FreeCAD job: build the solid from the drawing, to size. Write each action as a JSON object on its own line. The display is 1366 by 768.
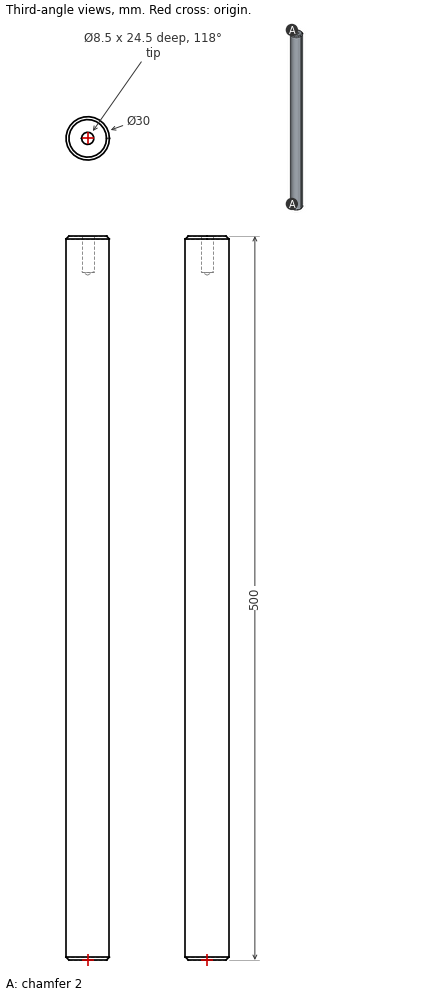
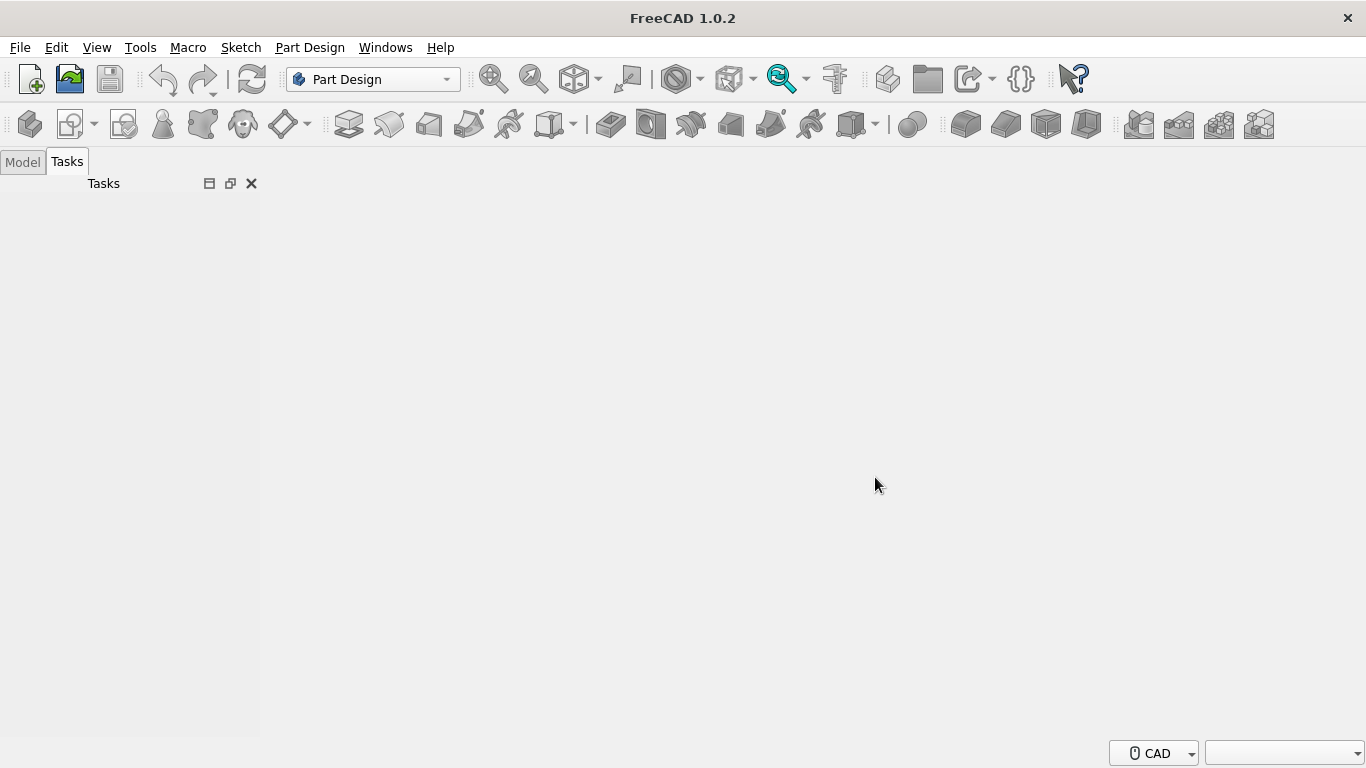
{"action": "left_click", "coordinate": [30, 80]}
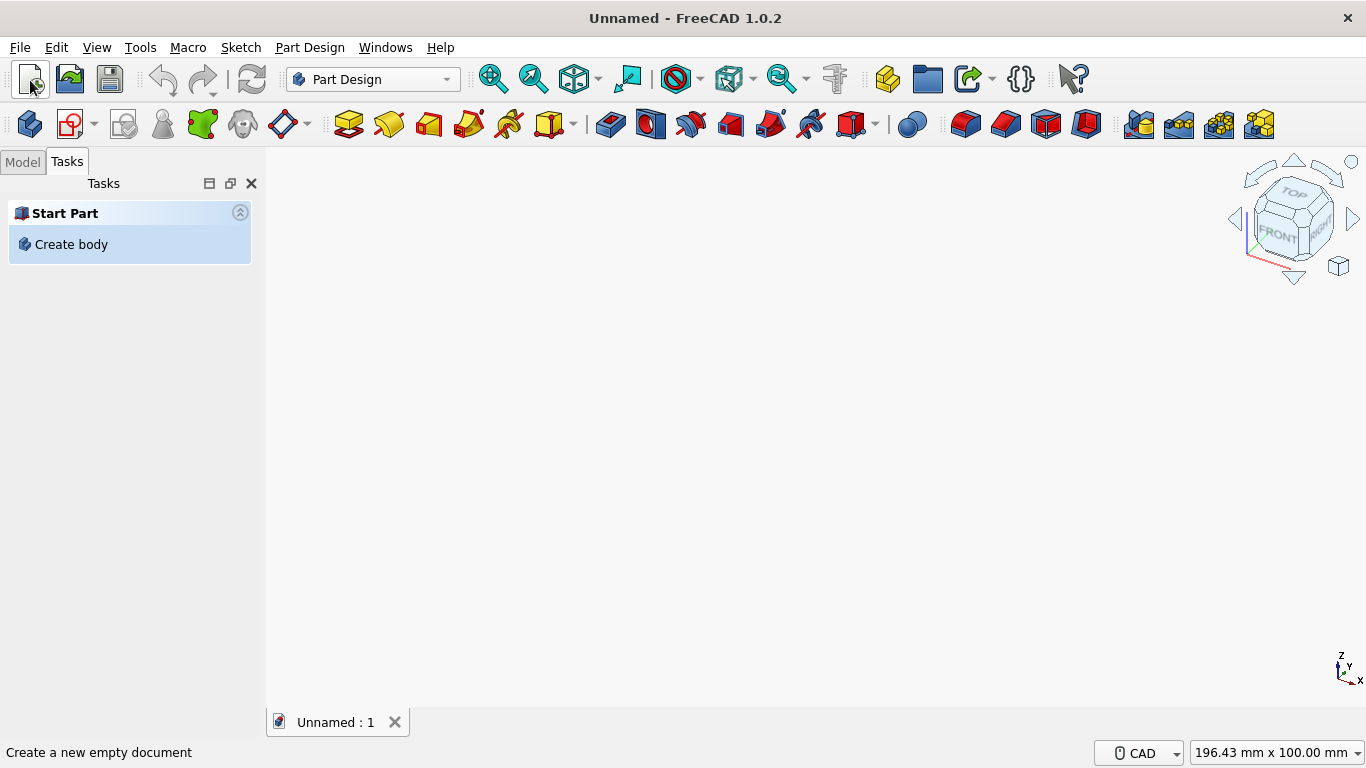
{"action": "left_click", "coordinate": [70, 124]}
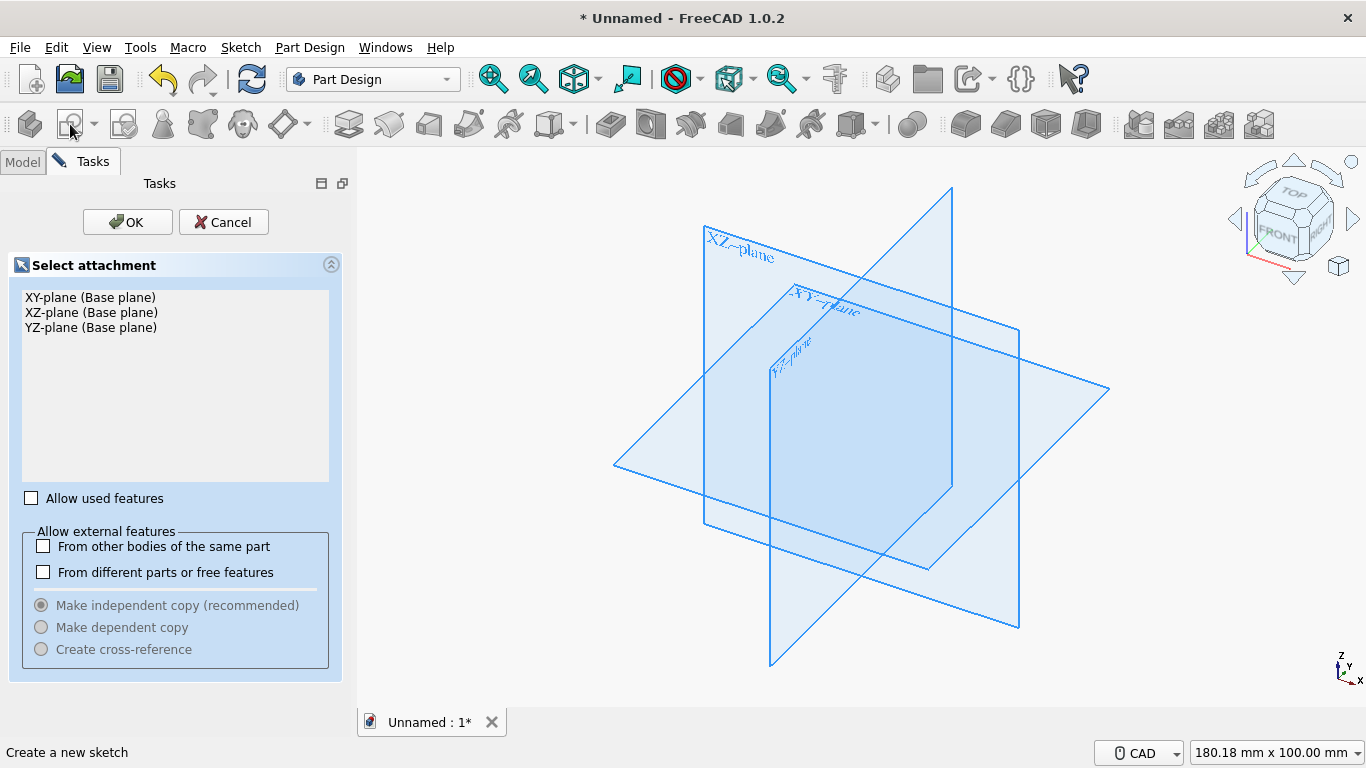
{"action": "left_click", "coordinate": [82, 298]}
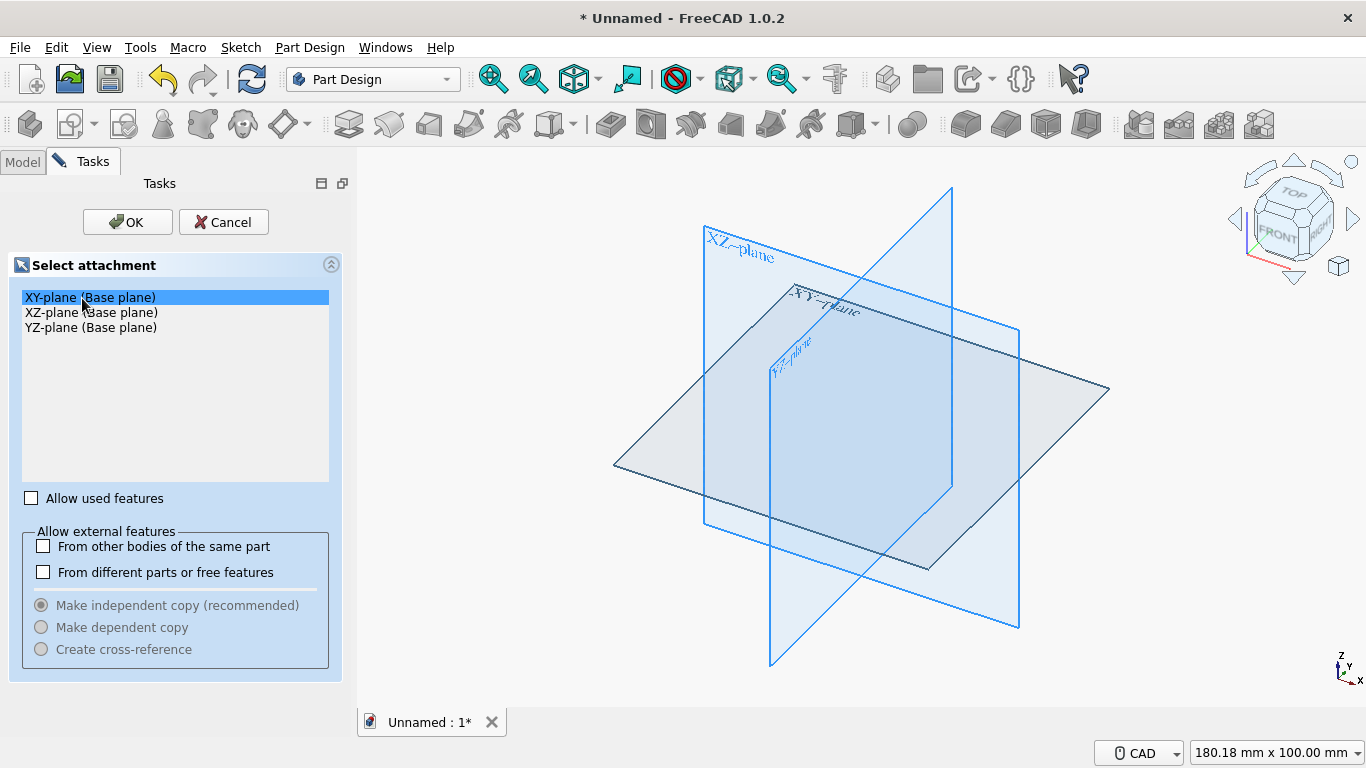
{"action": "left_click", "coordinate": [128, 222]}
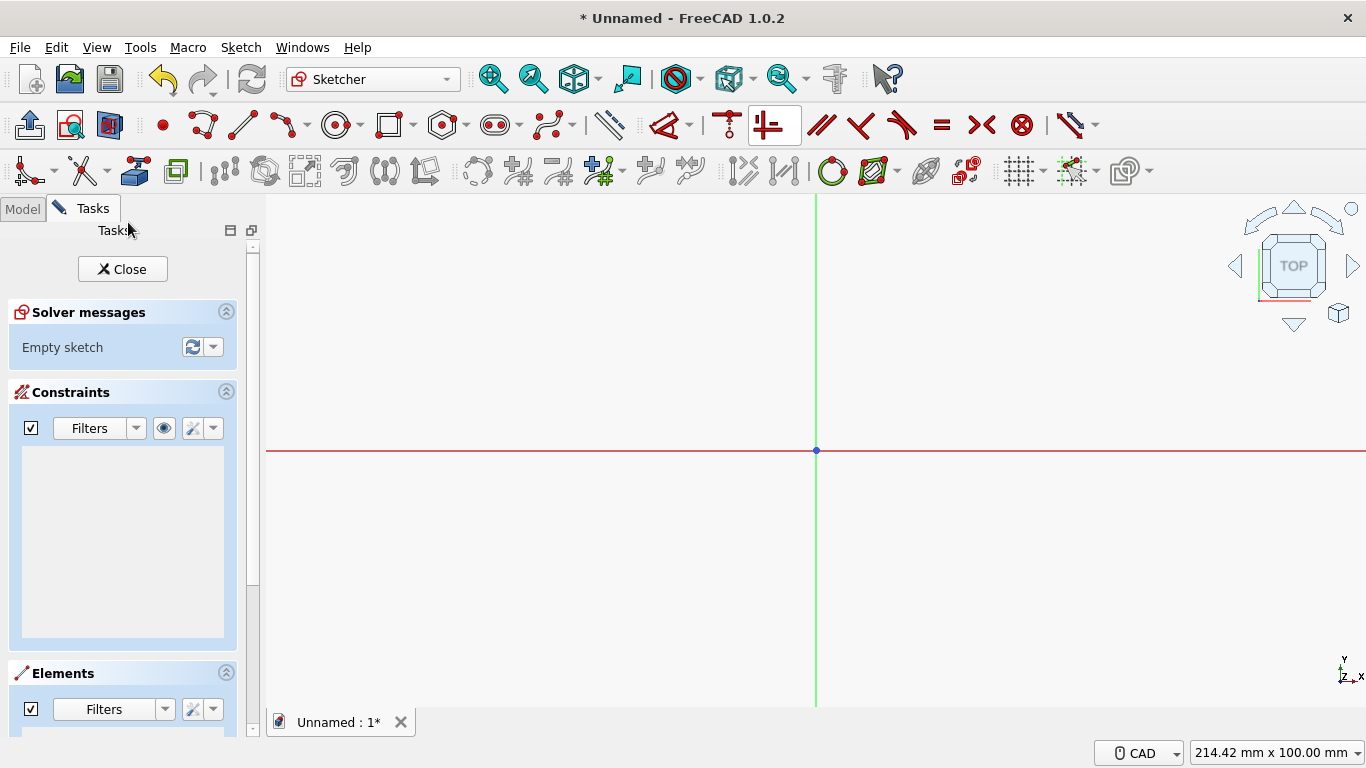
{"action": "scroll", "coordinate": [872, 450], "scroll_direction": "up", "scroll_amount": 4}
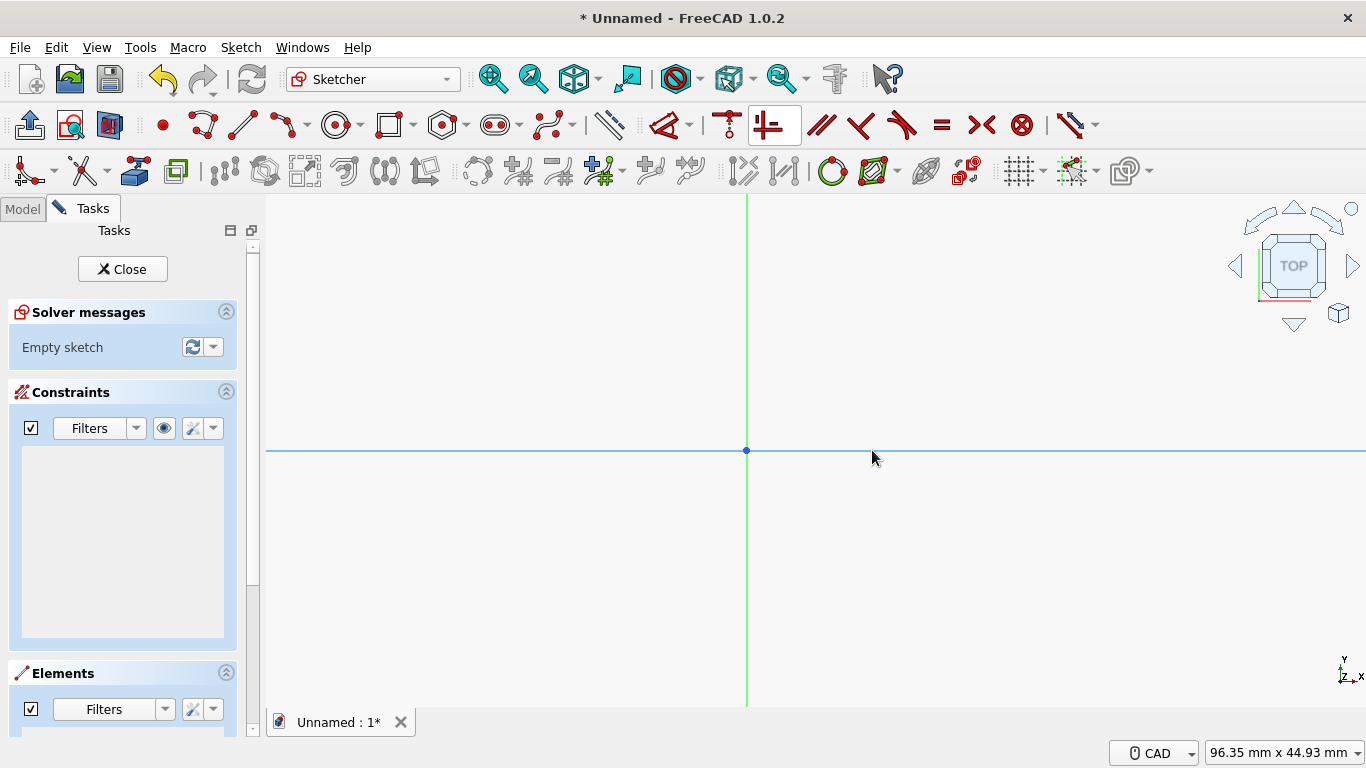
{"action": "left_click", "coordinate": [336, 126]}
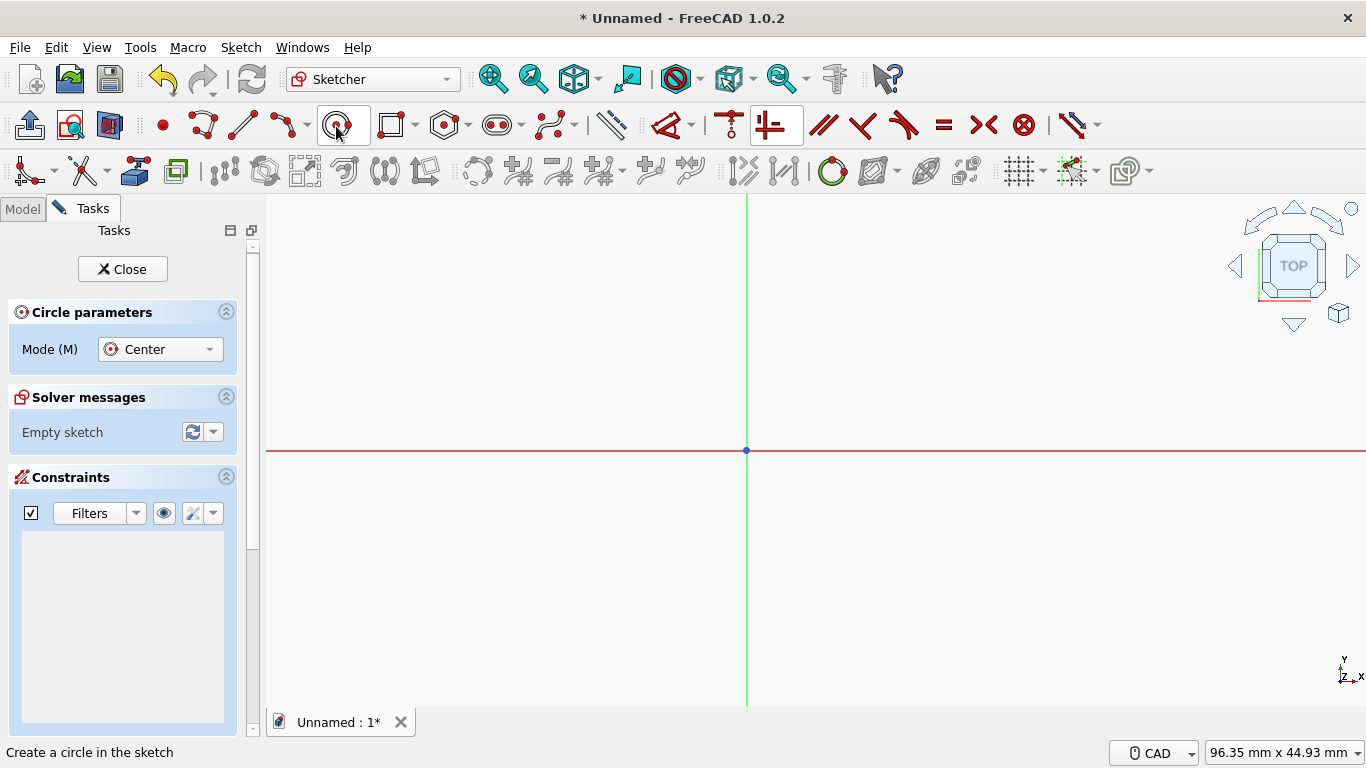
{"action": "left_click", "coordinate": [747, 450]}
{"action": "left_click", "coordinate": [868, 329]}
{"action": "key", "text": "Escape"}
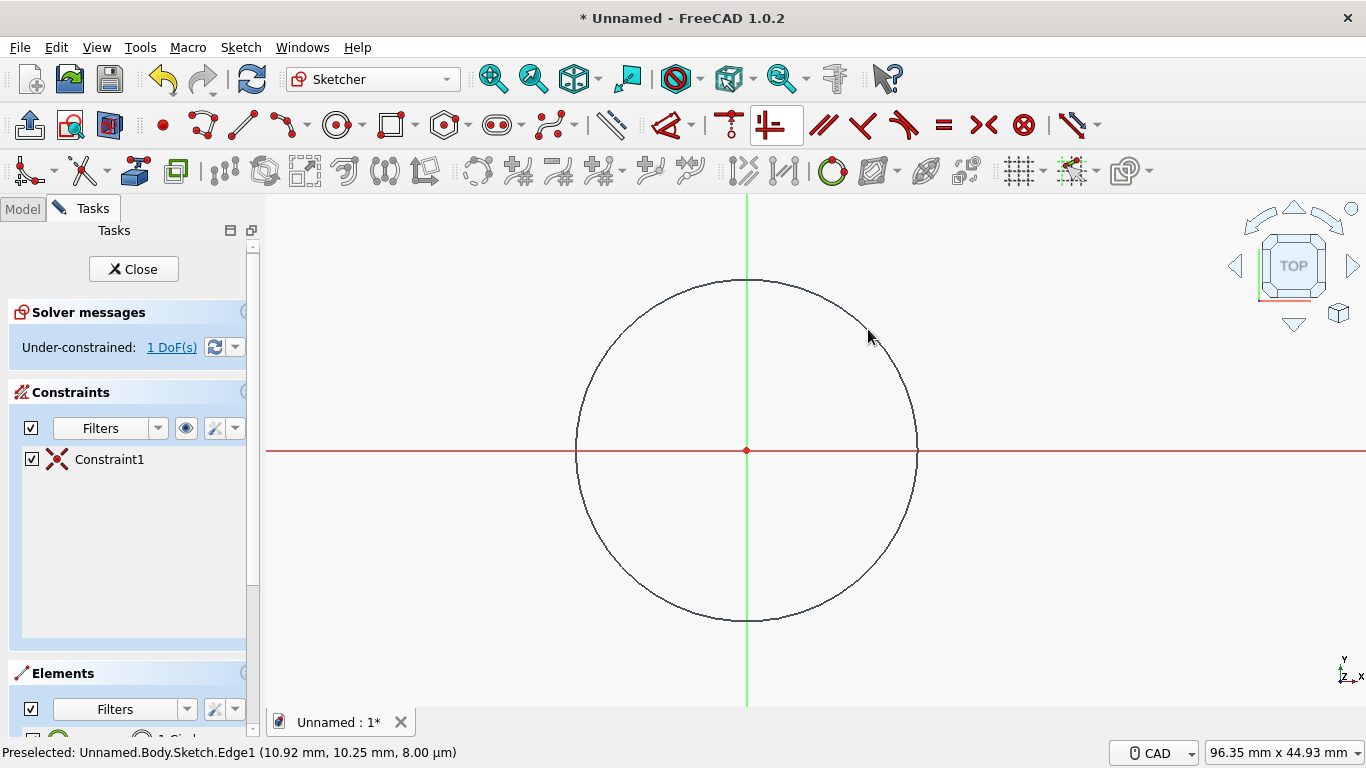
{"action": "key", "text": "d"}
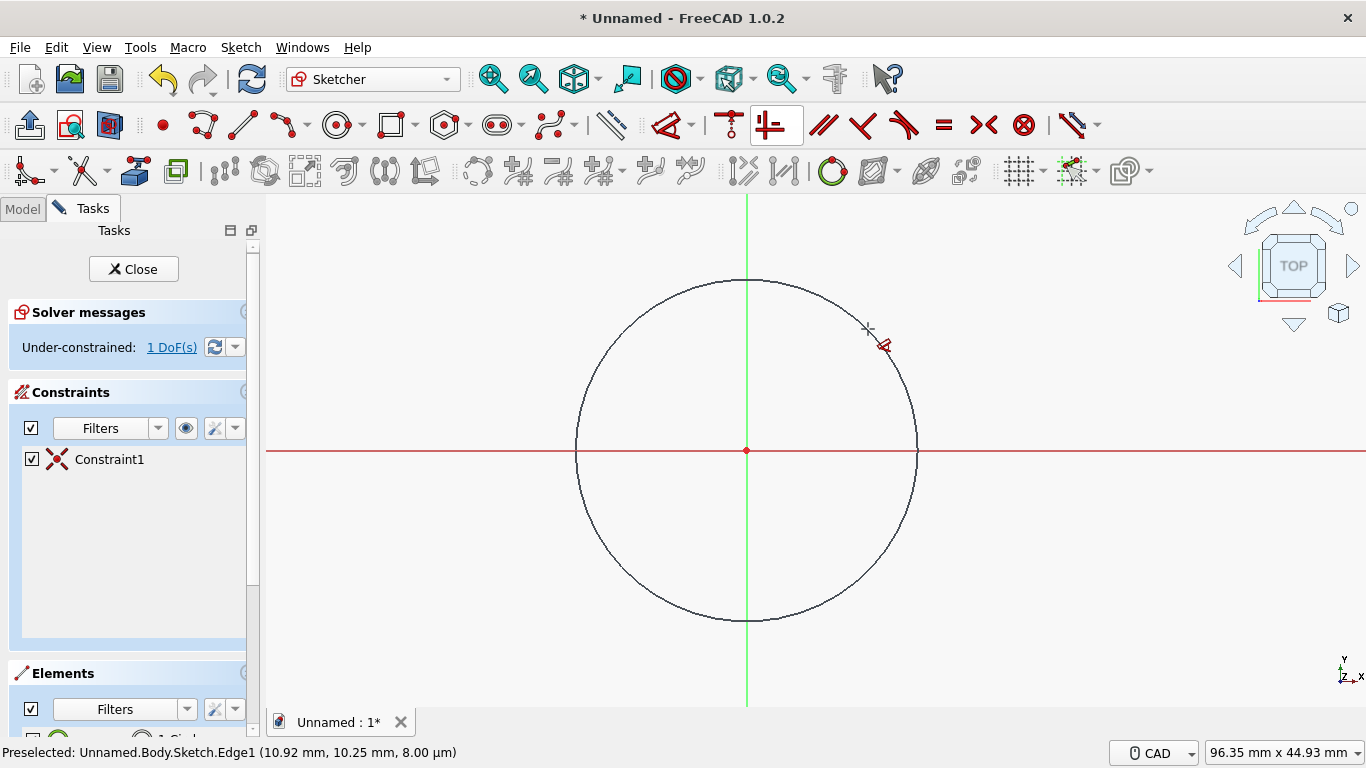
{"action": "left_click", "coordinate": [867, 329]}
{"action": "left_click", "coordinate": [890, 306]}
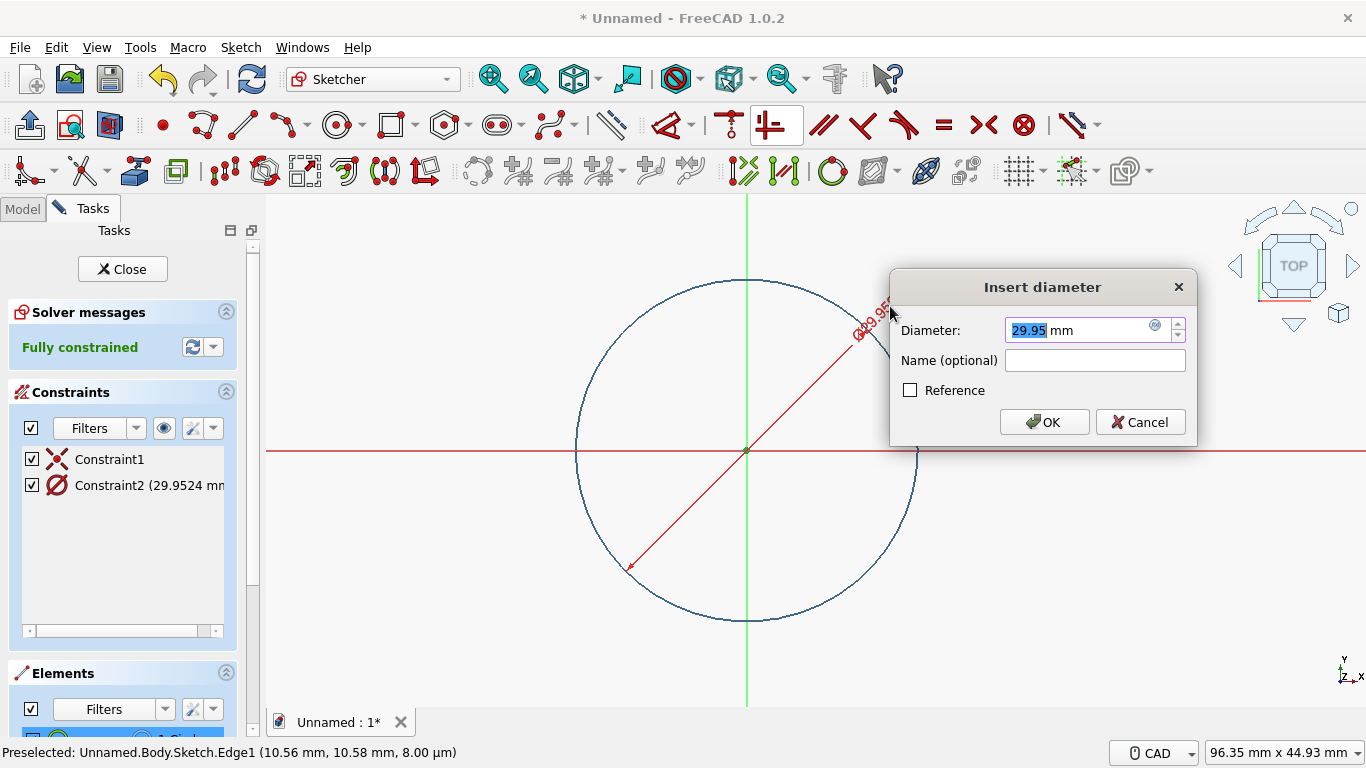
{"action": "type", "text": "30"}
{"action": "key", "text": "Return"}
{"action": "key", "text": "Escape"}